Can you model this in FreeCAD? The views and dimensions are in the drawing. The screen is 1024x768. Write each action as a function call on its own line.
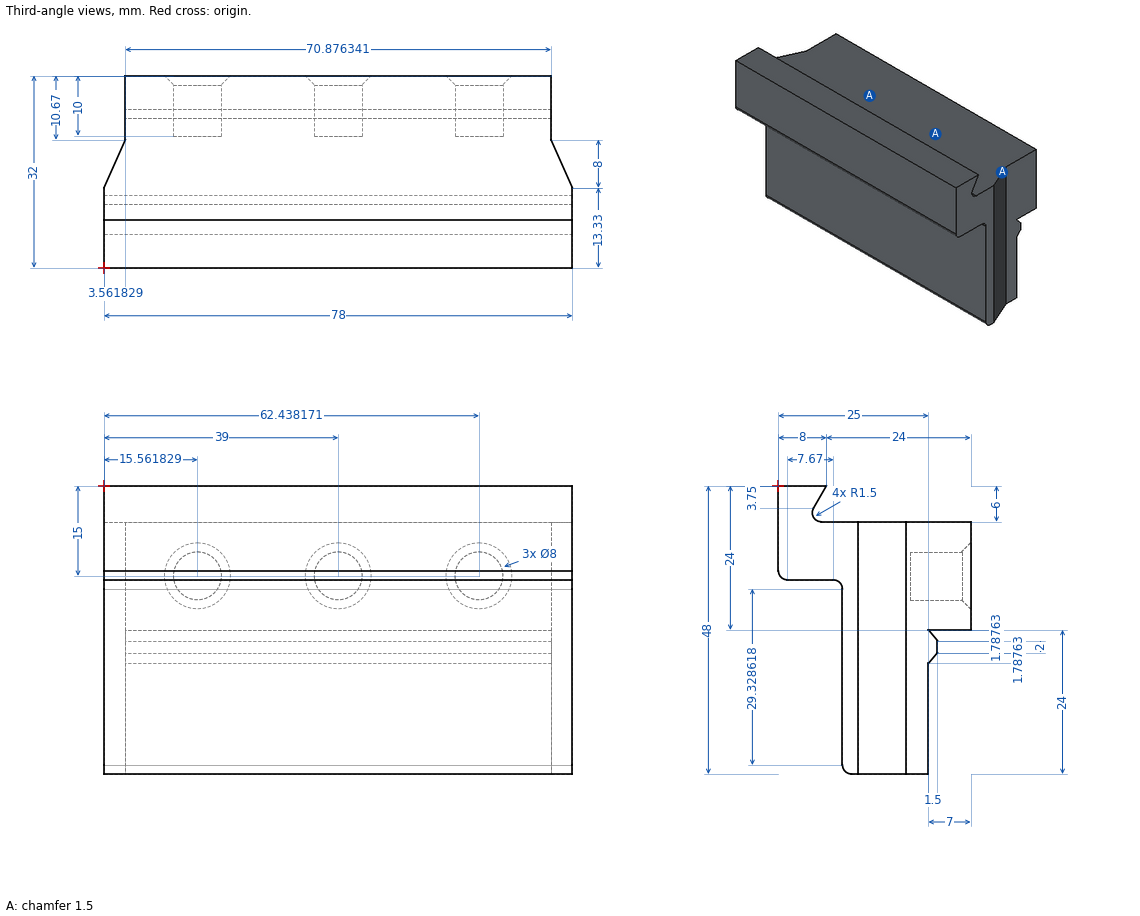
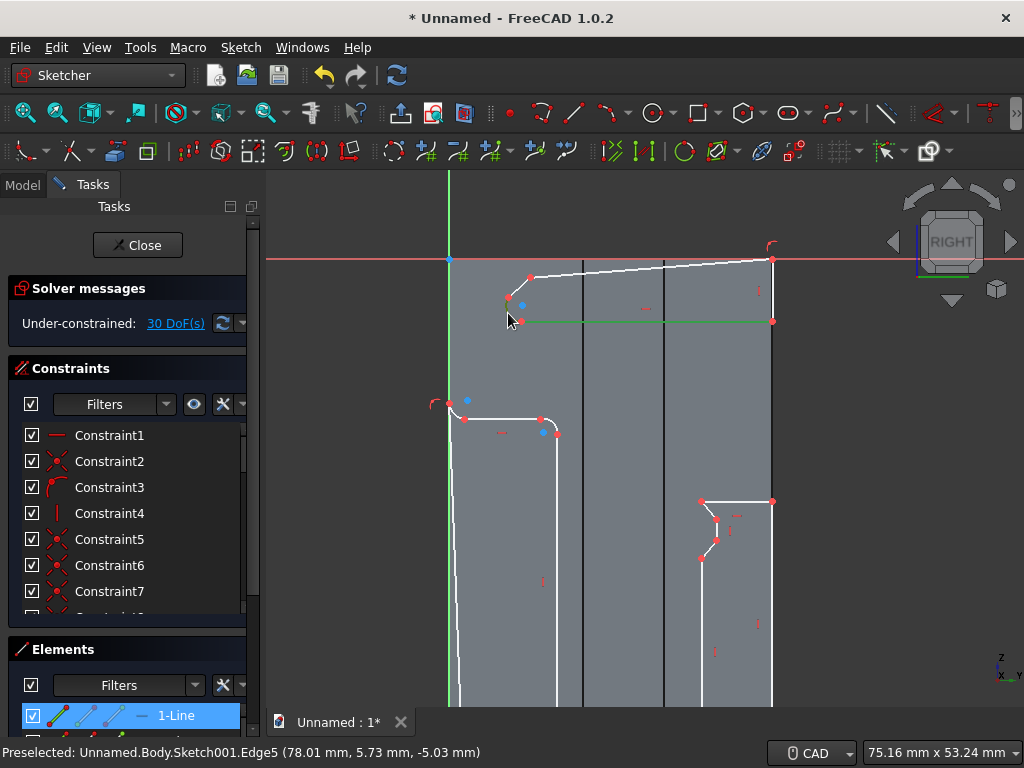
key(t)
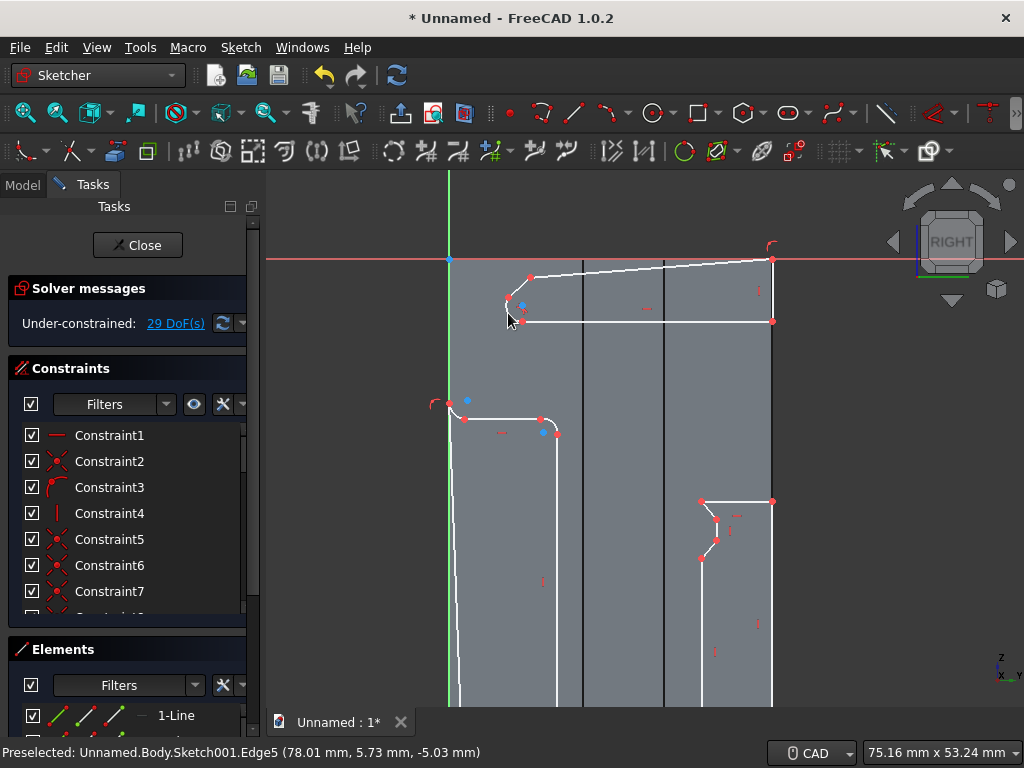
click(522, 286)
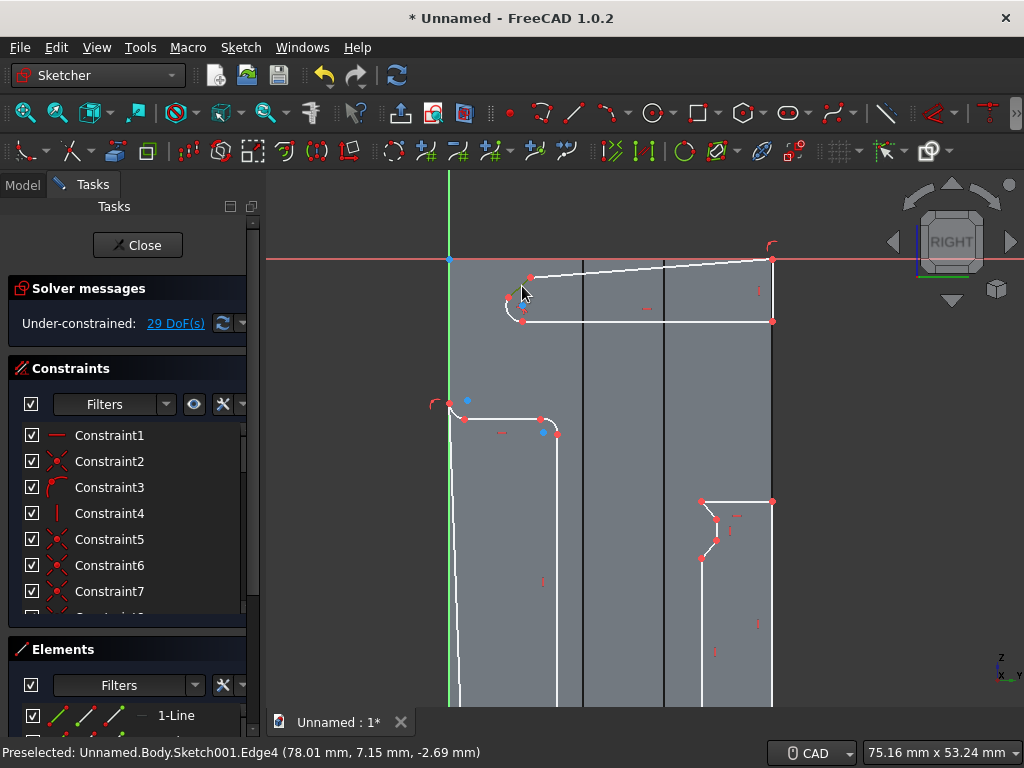
scroll(506, 307, up, 2)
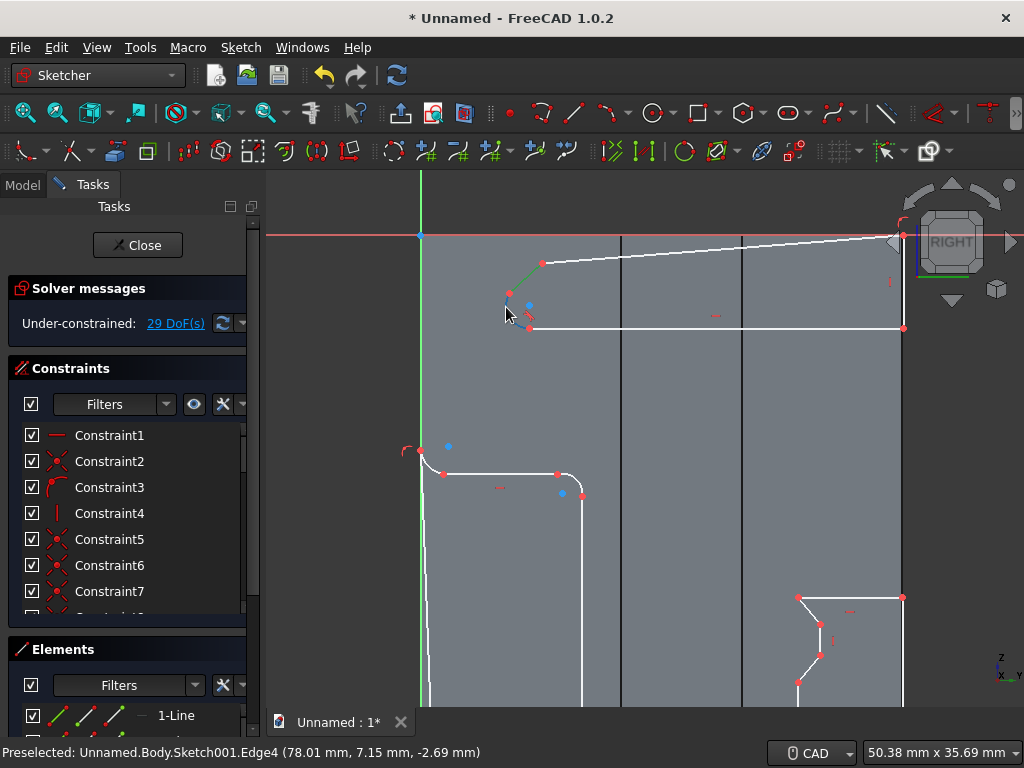
click(506, 308)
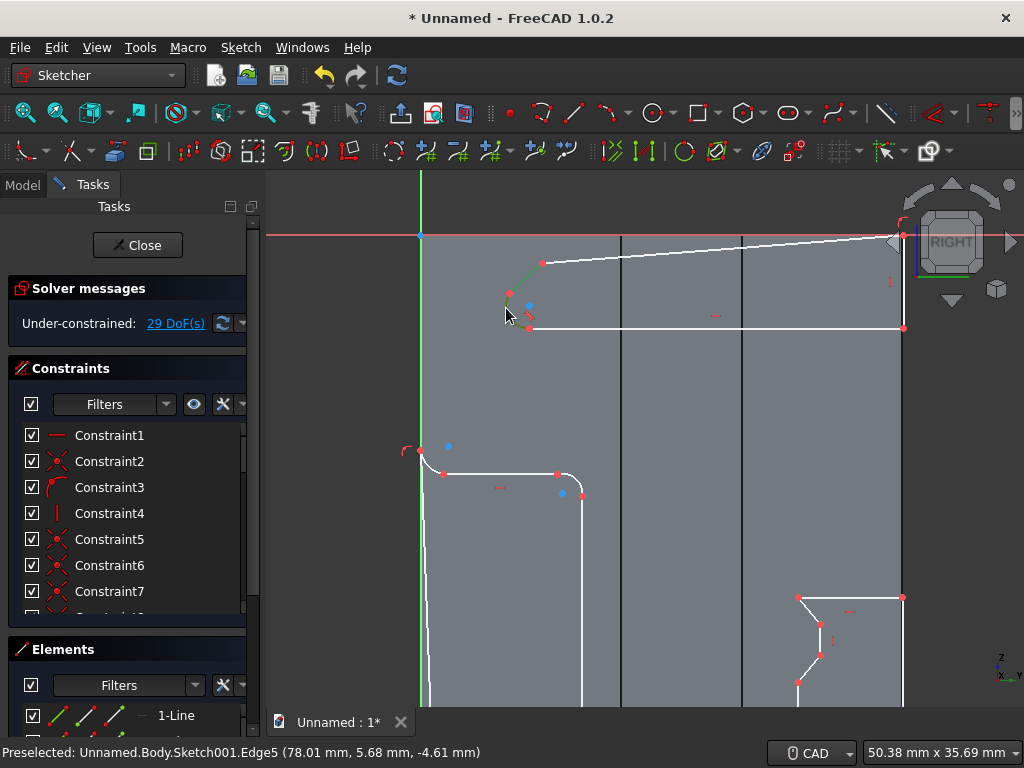
key(t)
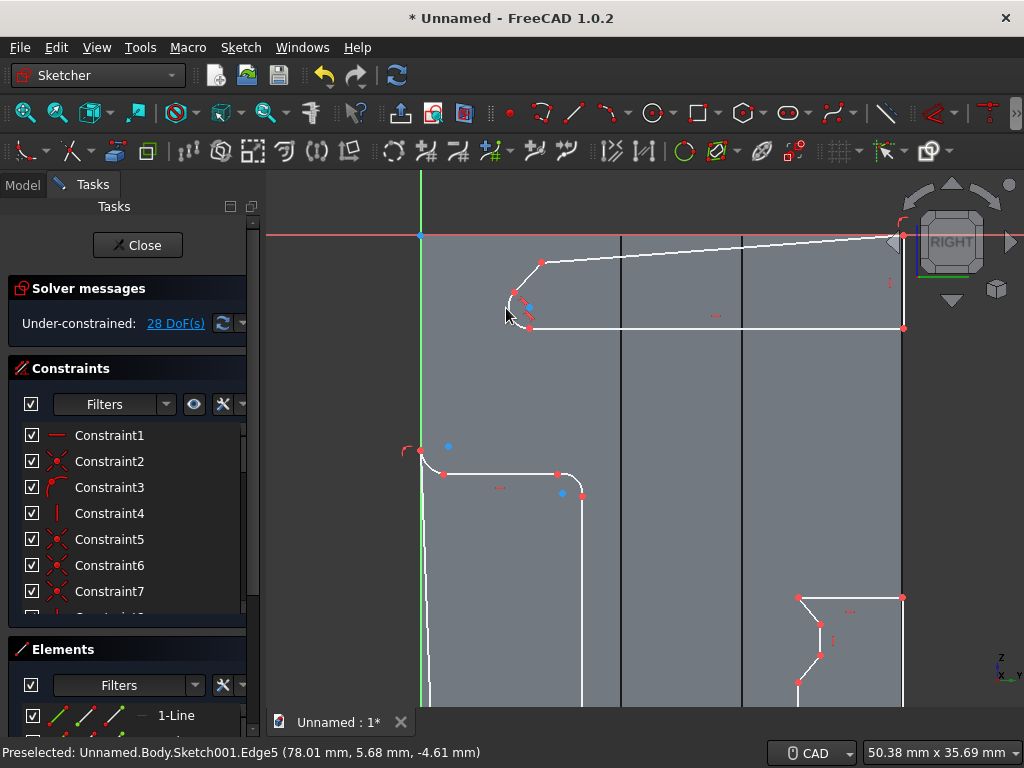
click(582, 629)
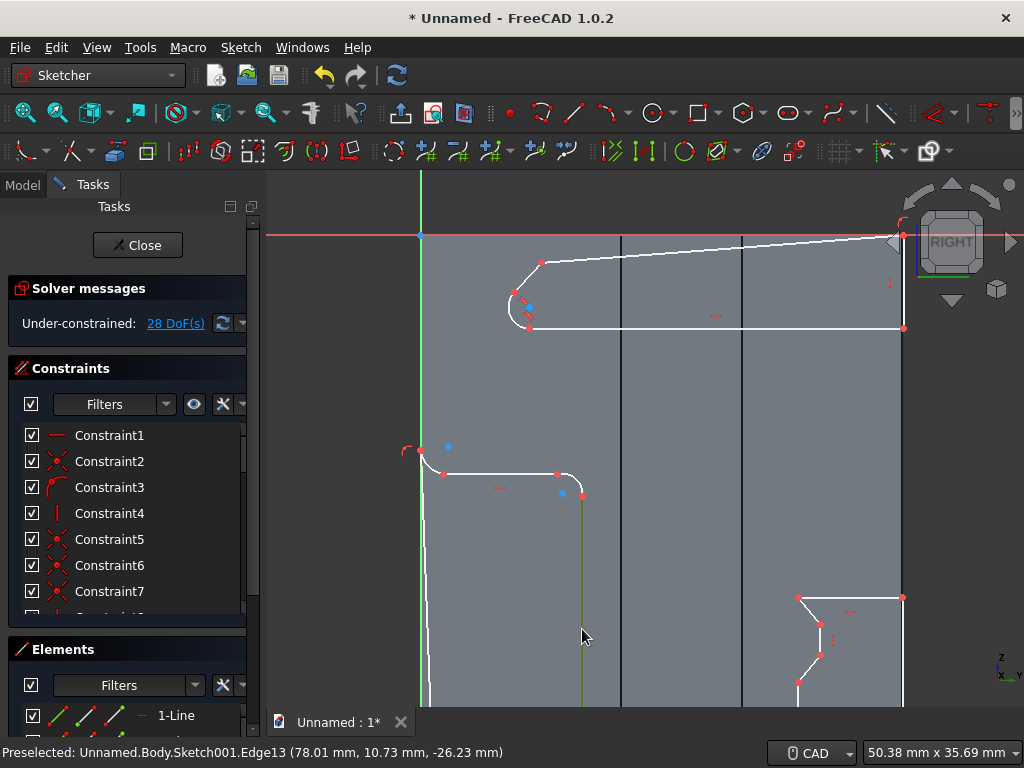
click(580, 485)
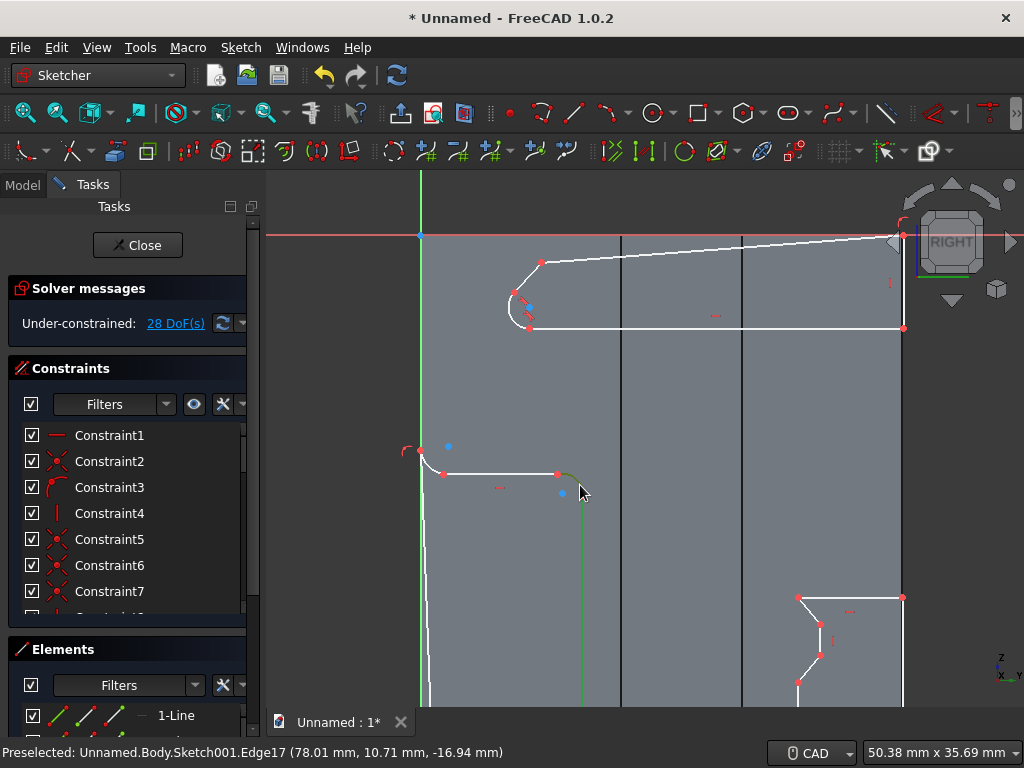
key(t)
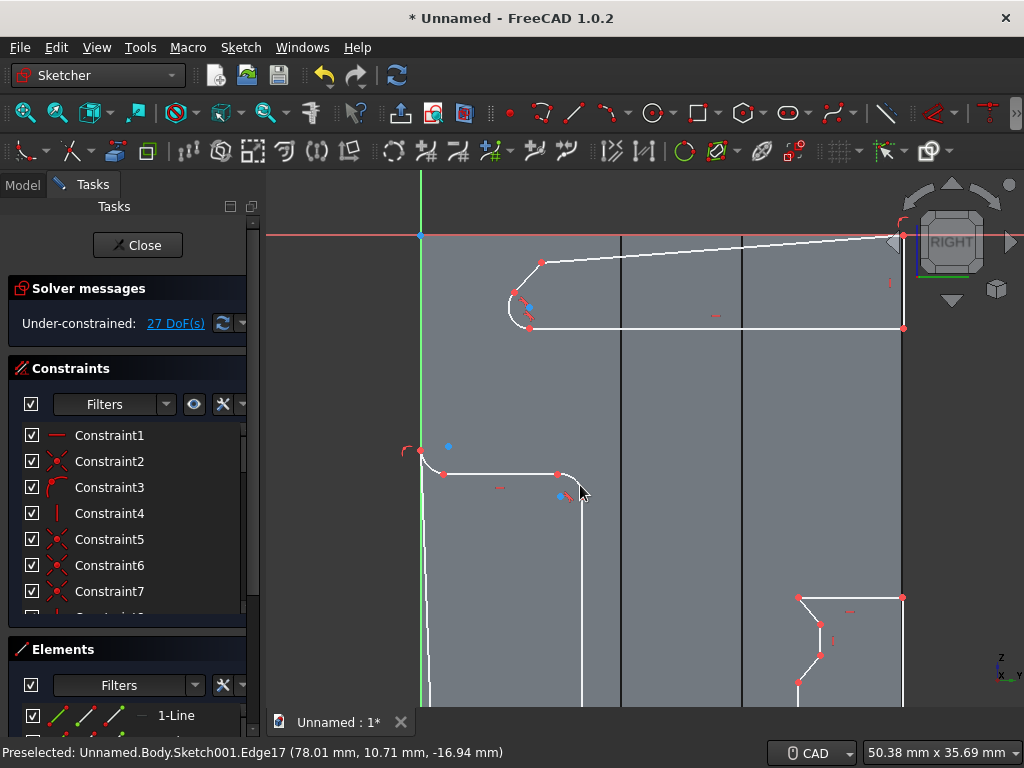
click(582, 628)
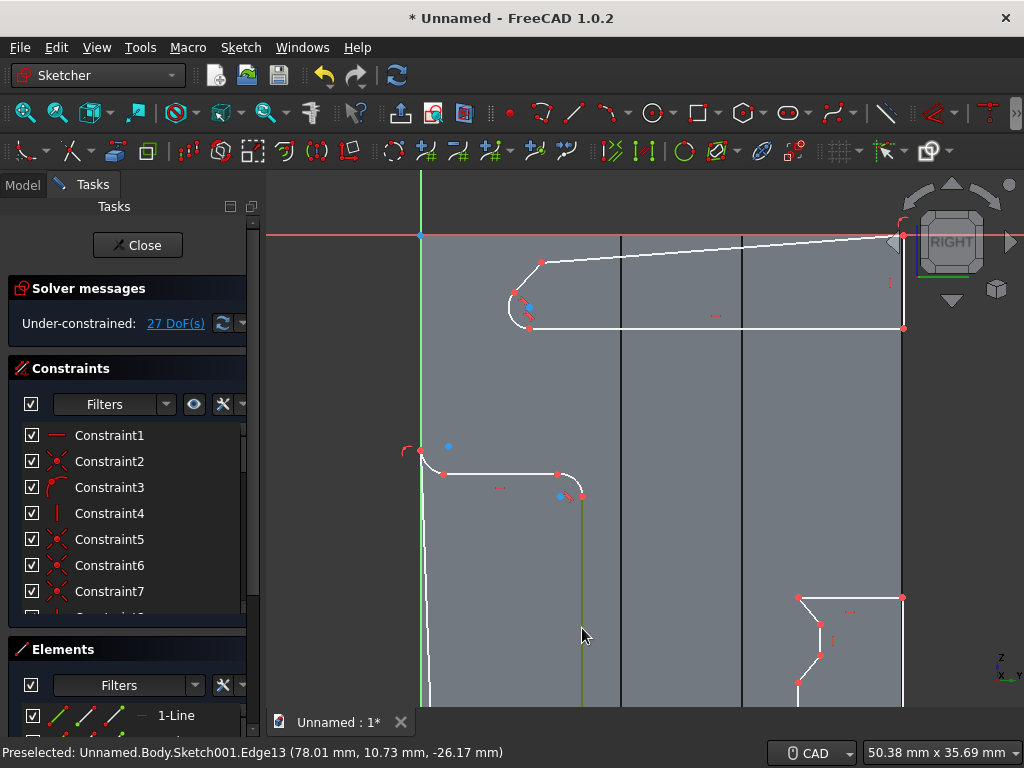
scroll(507, 310, down, 4)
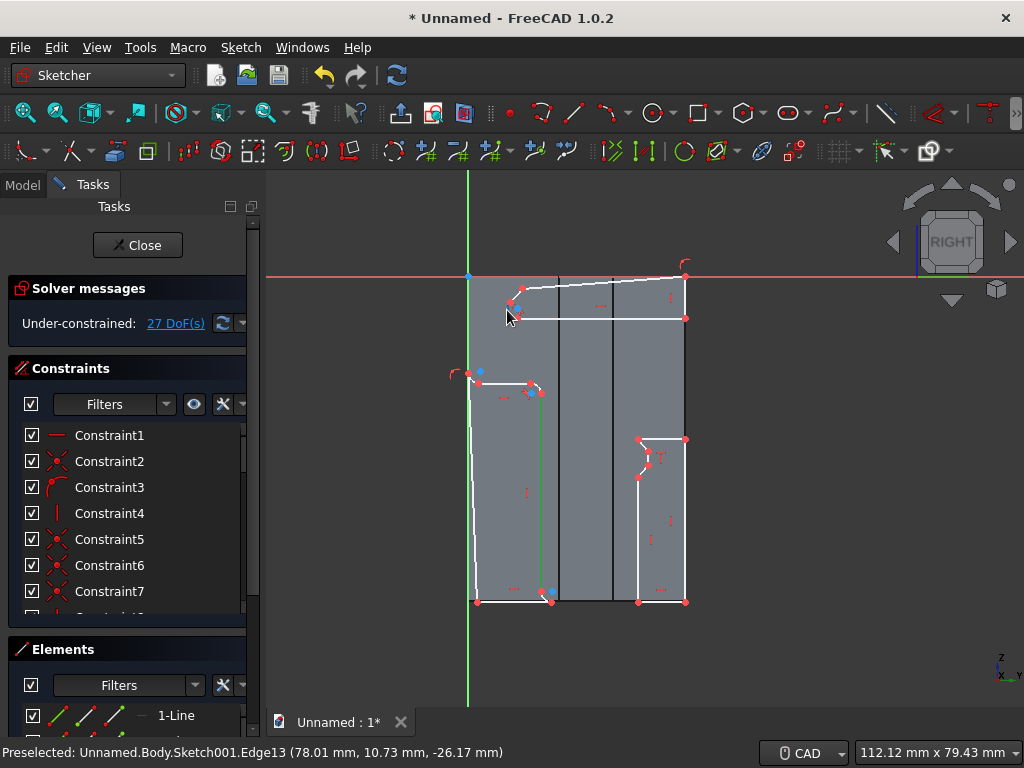
scroll(542, 596, up, 6)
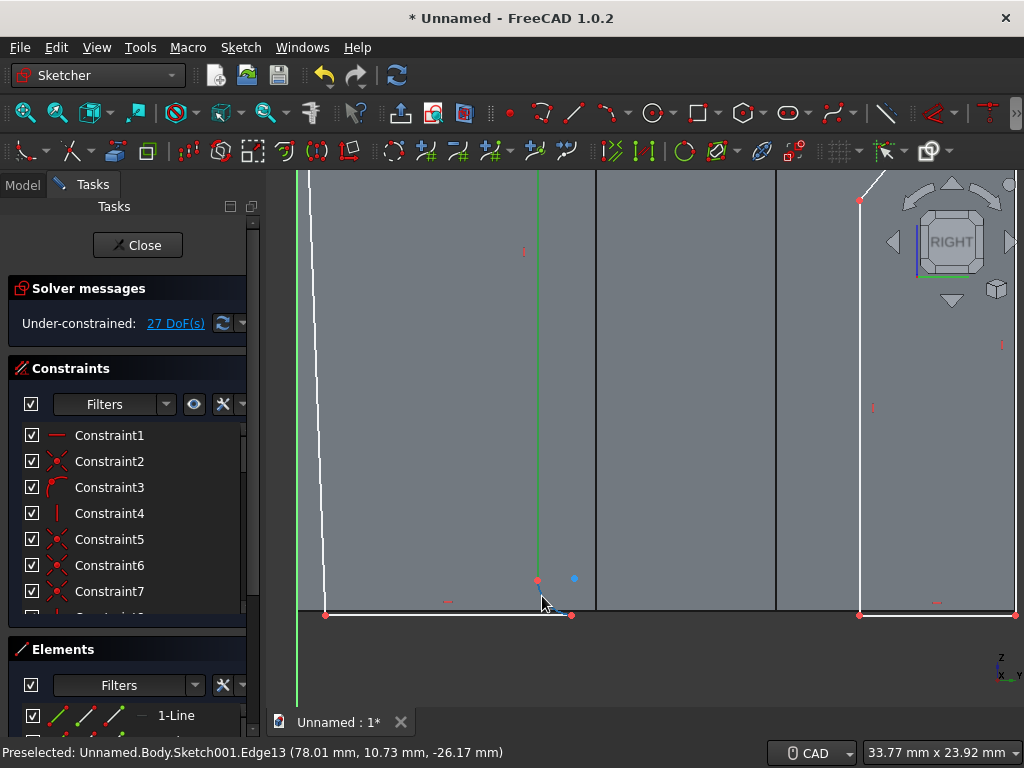
click(542, 595)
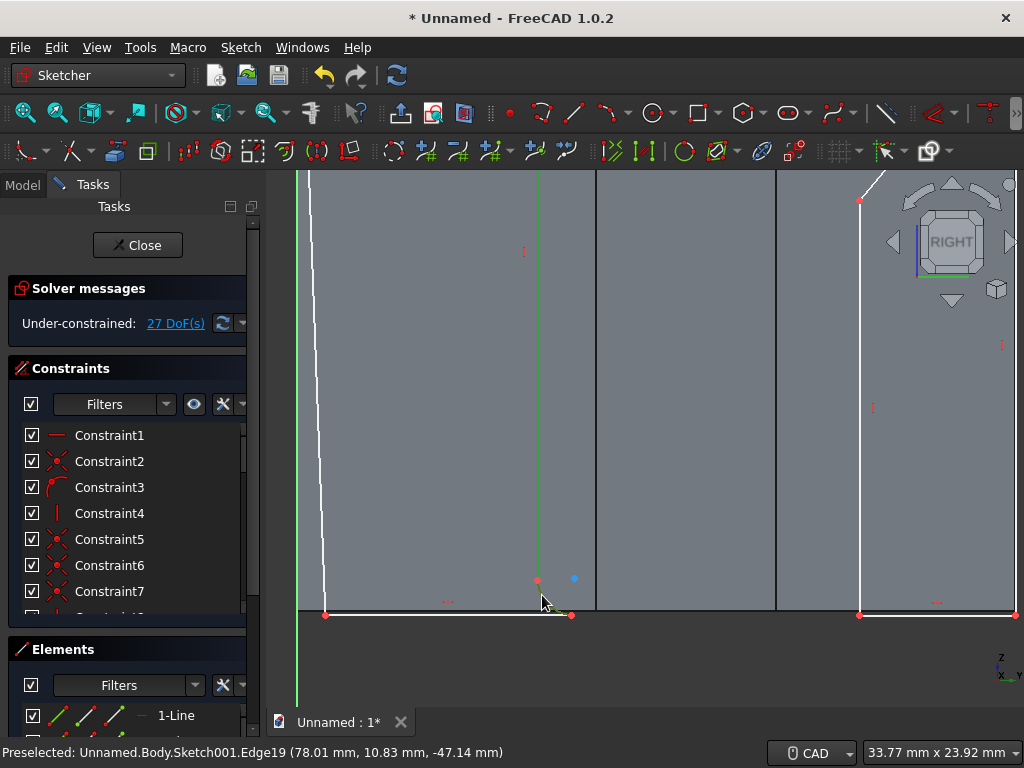
key(t)